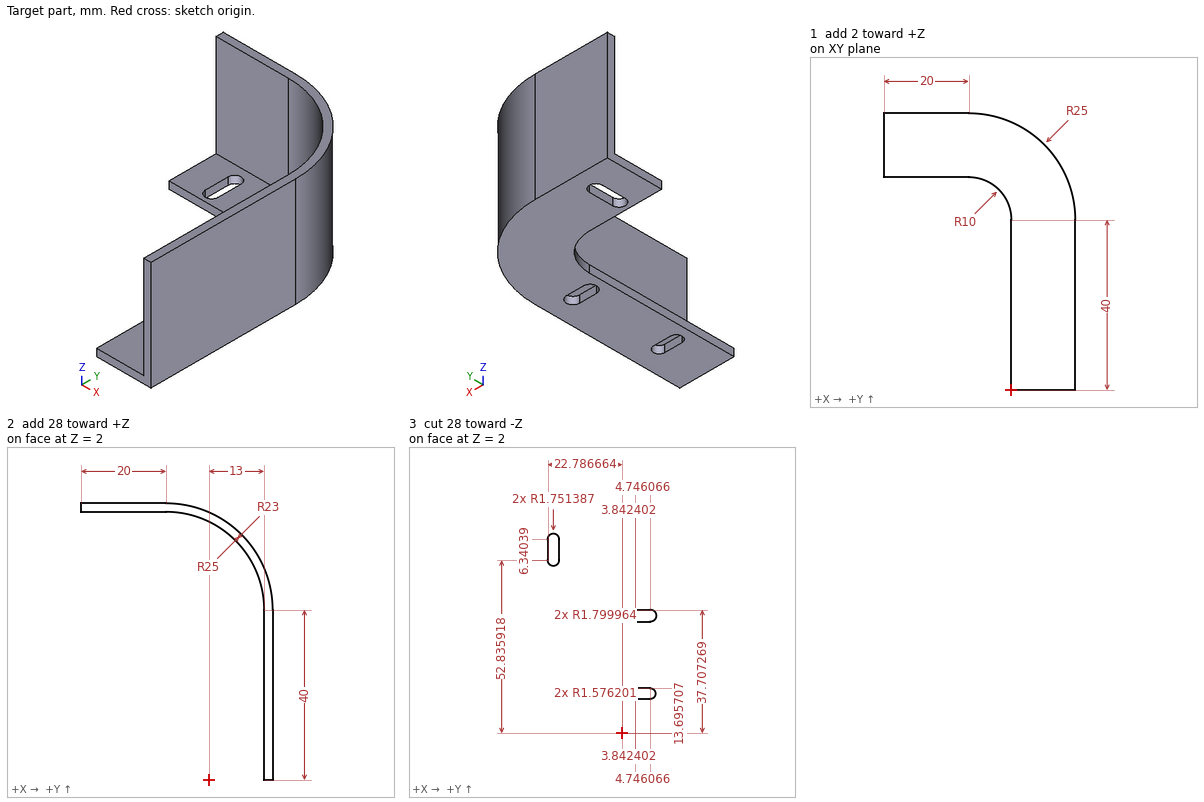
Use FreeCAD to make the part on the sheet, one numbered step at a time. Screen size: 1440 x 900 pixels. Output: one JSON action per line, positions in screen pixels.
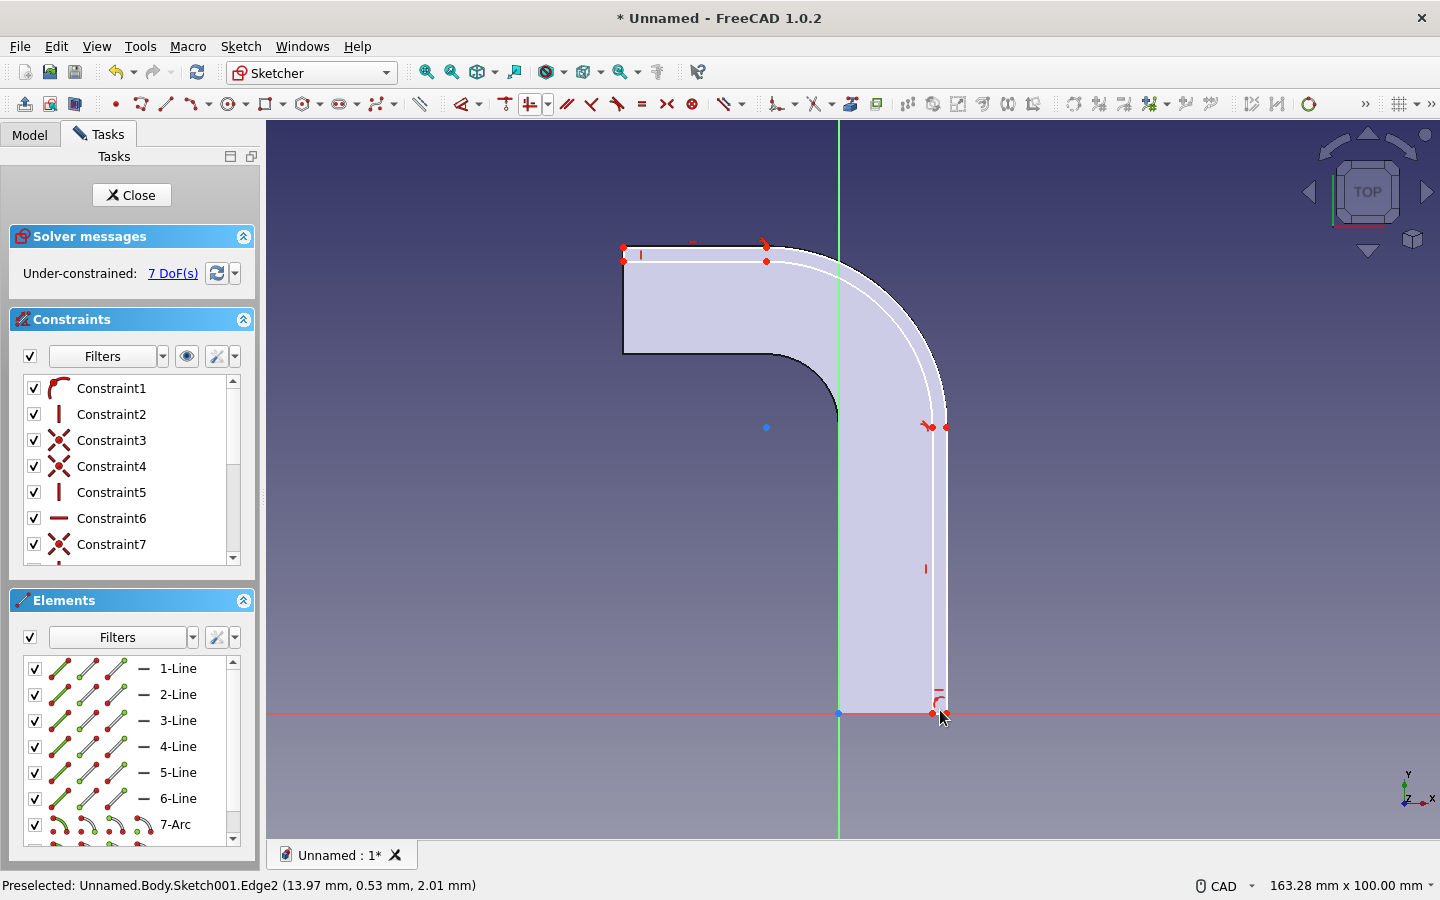
{"action": "left_click", "coordinate": [927, 346]}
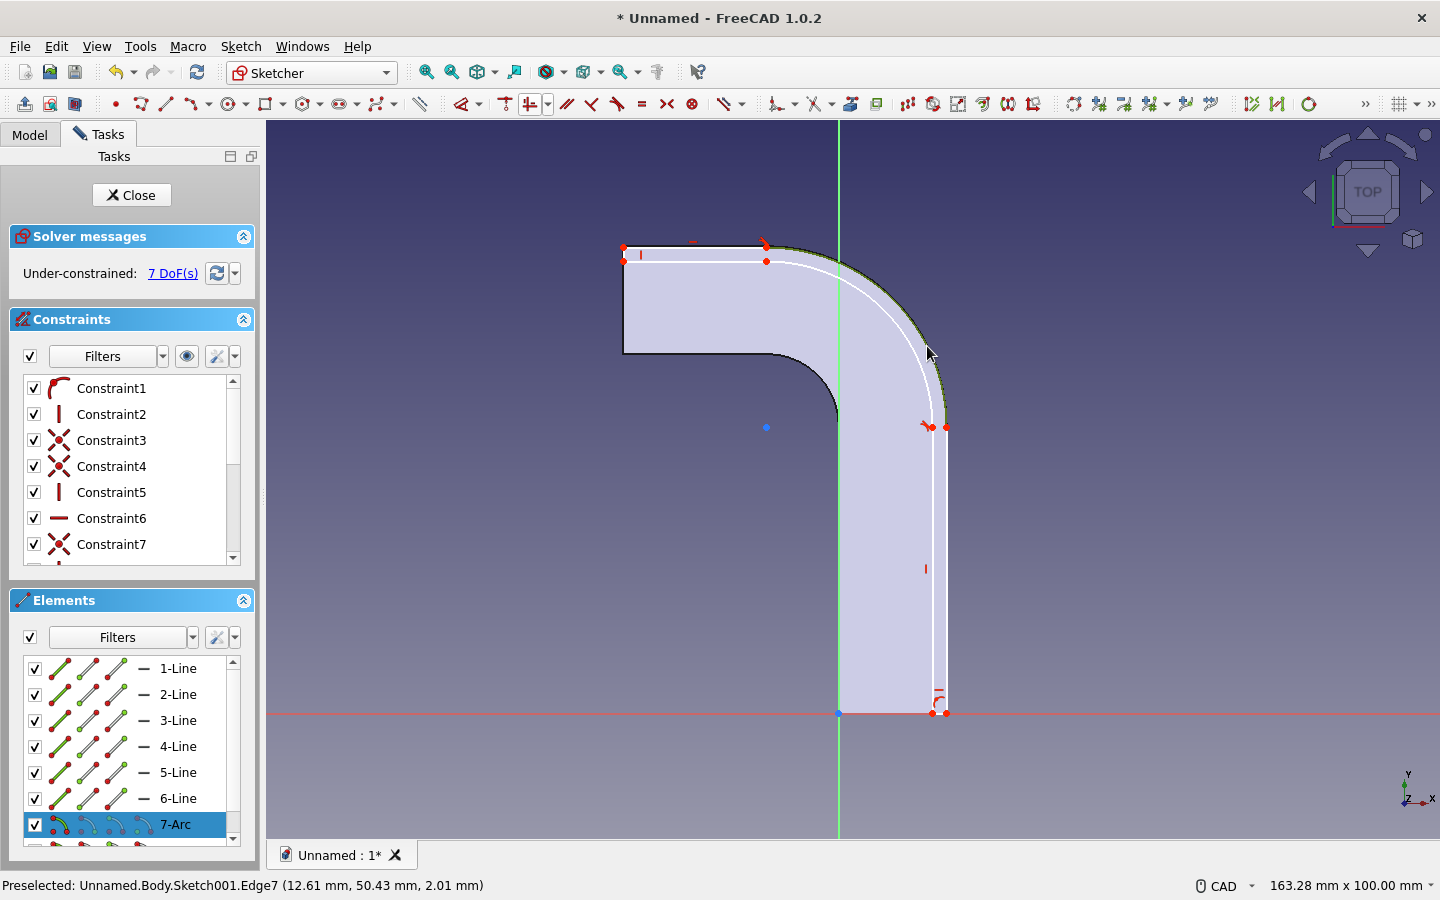
{"action": "left_click", "coordinate": [914, 352]}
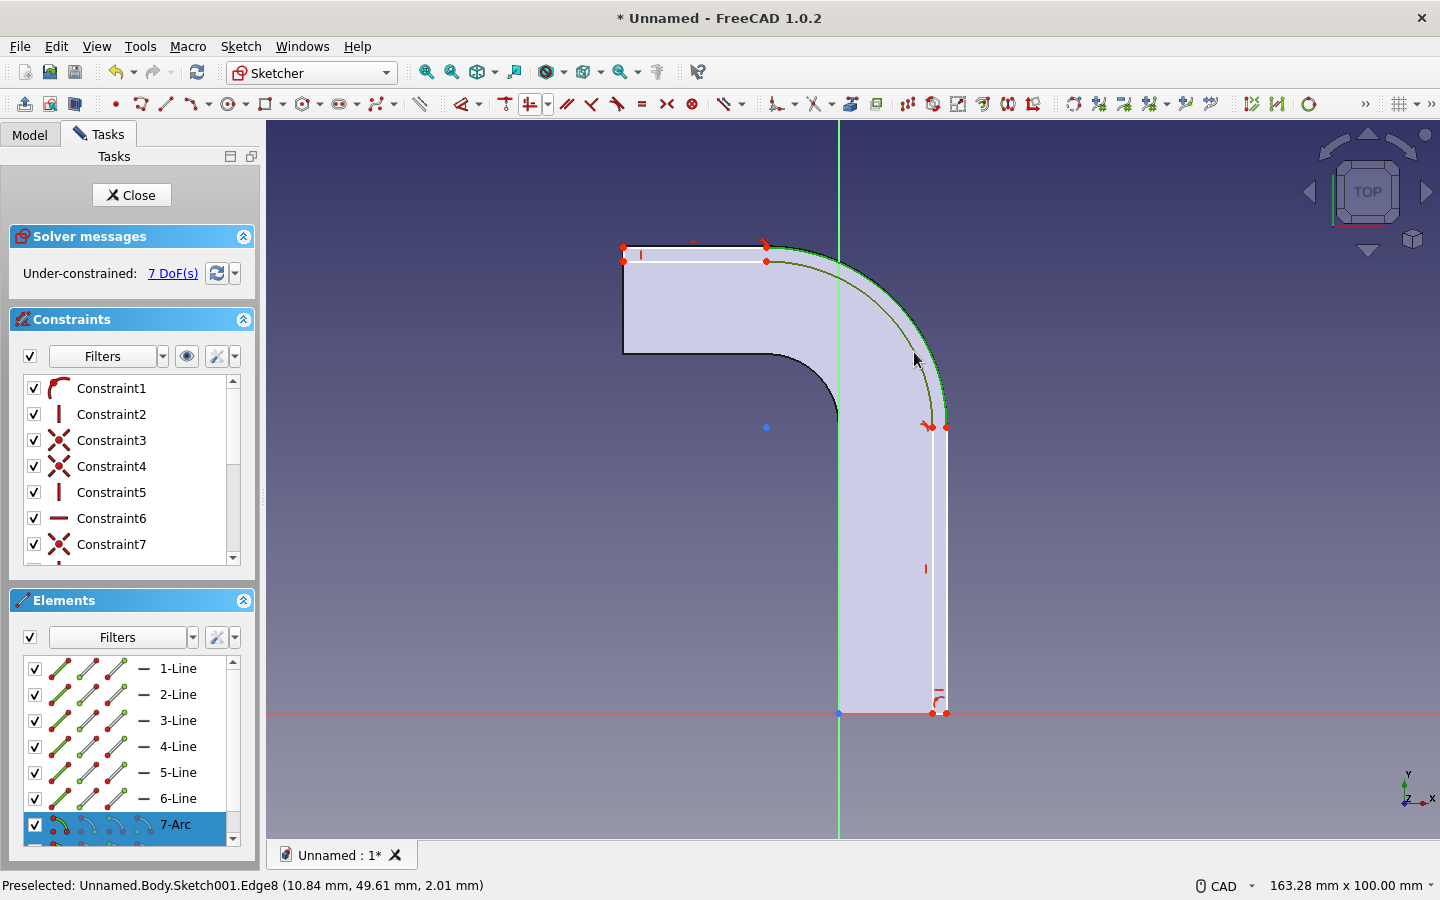
{"action": "left_click", "coordinate": [505, 104]}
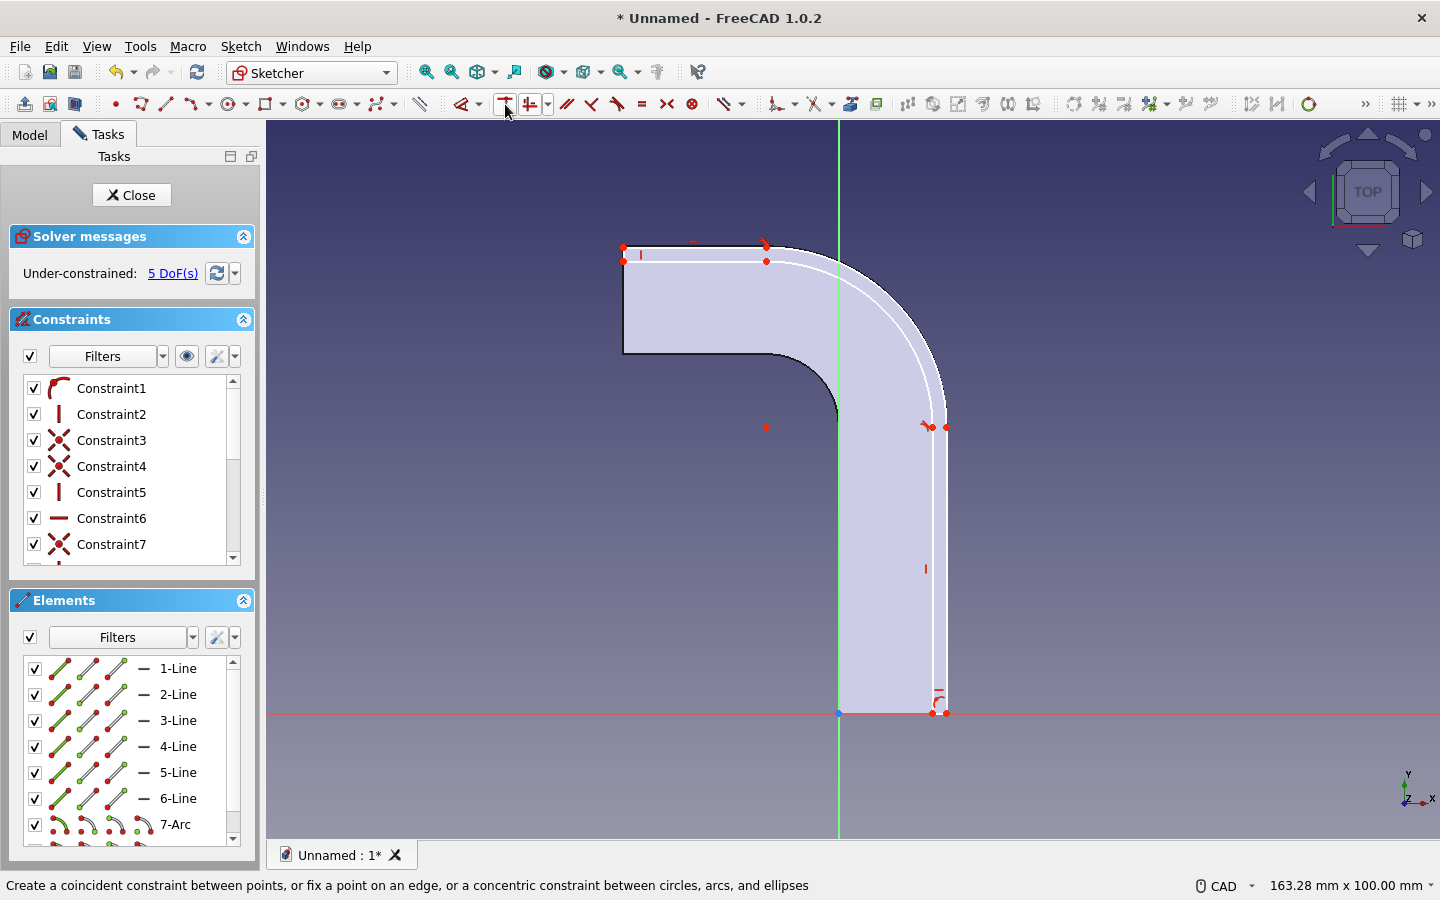
{"action": "left_click", "coordinate": [460, 104]}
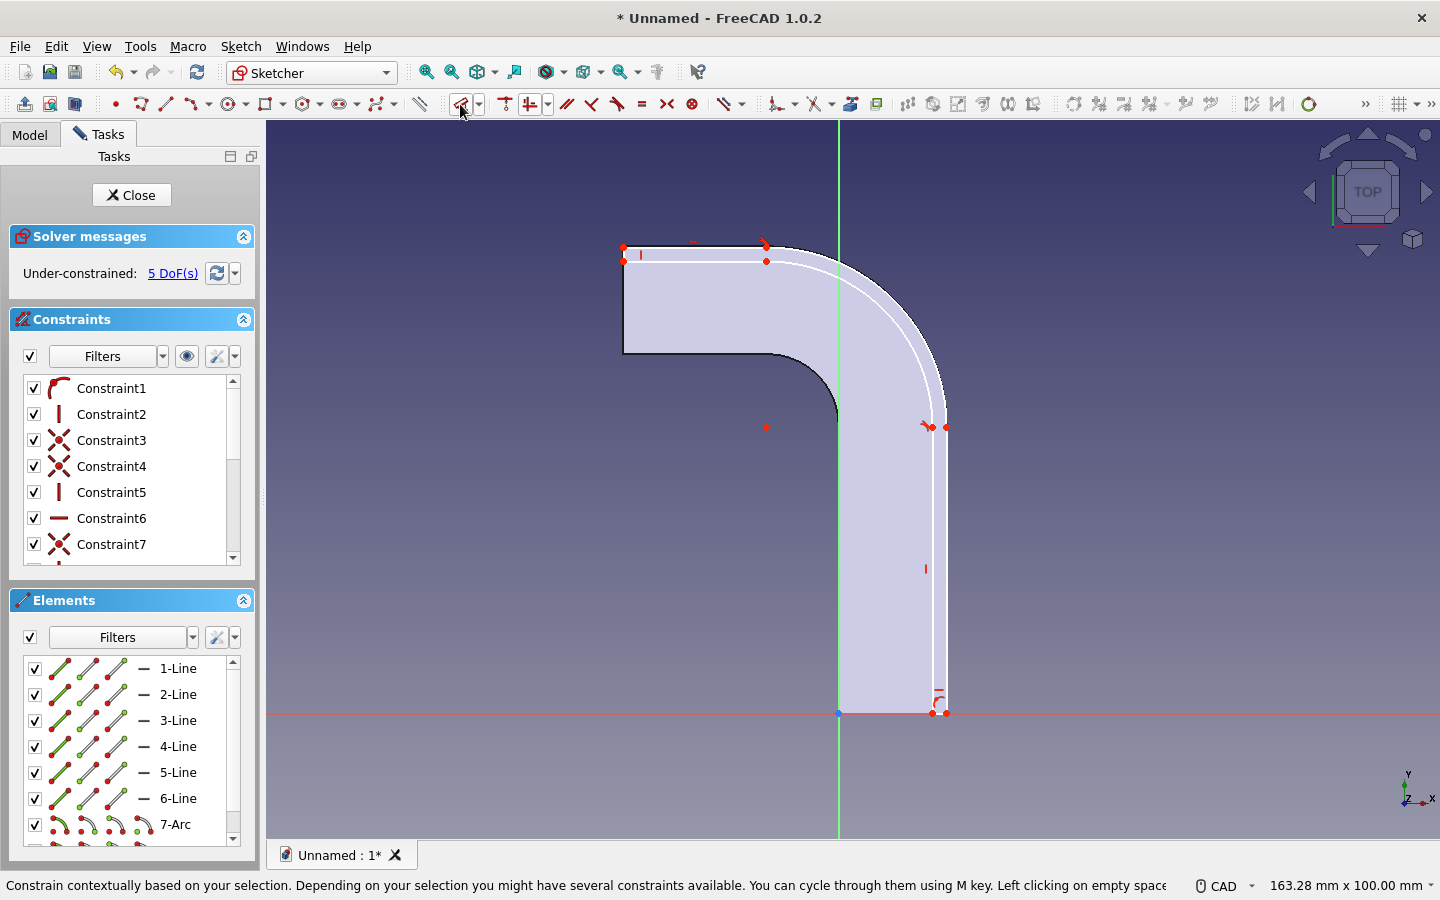
{"action": "left_click", "coordinate": [927, 346]}
{"action": "left_click", "coordinate": [956, 332]}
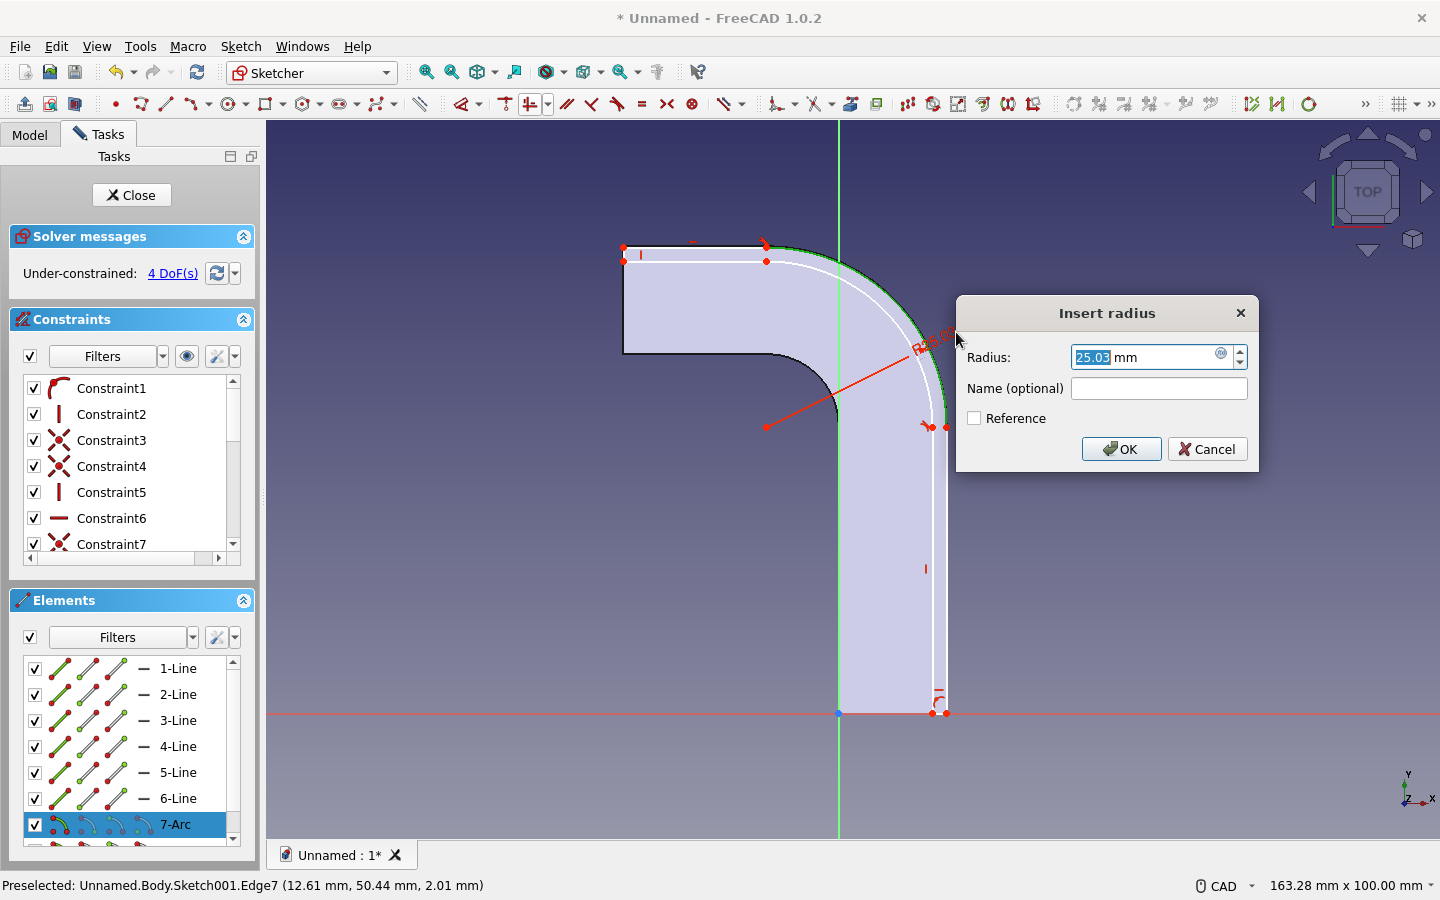
{"action": "type", "text": "25"}
{"action": "key", "text": "Return"}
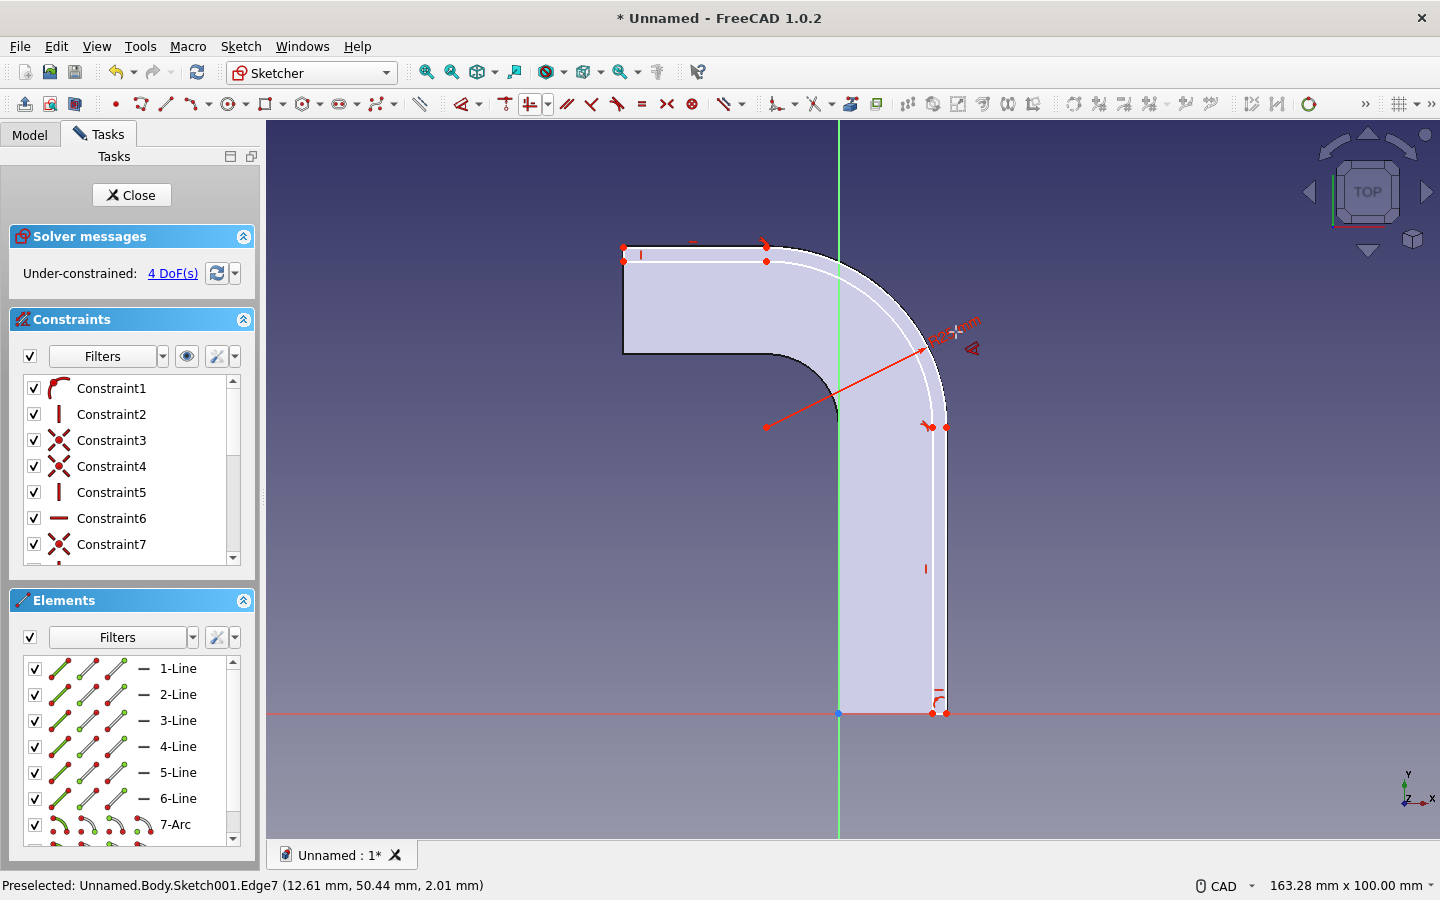
{"action": "left_click", "coordinate": [914, 352]}
{"action": "left_click", "coordinate": [964, 433]}